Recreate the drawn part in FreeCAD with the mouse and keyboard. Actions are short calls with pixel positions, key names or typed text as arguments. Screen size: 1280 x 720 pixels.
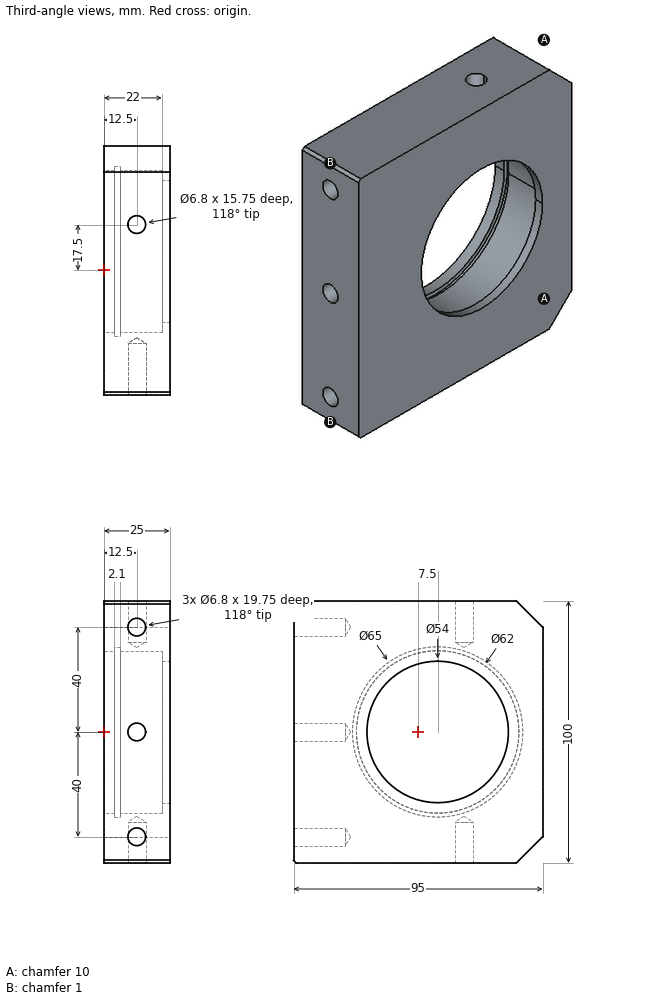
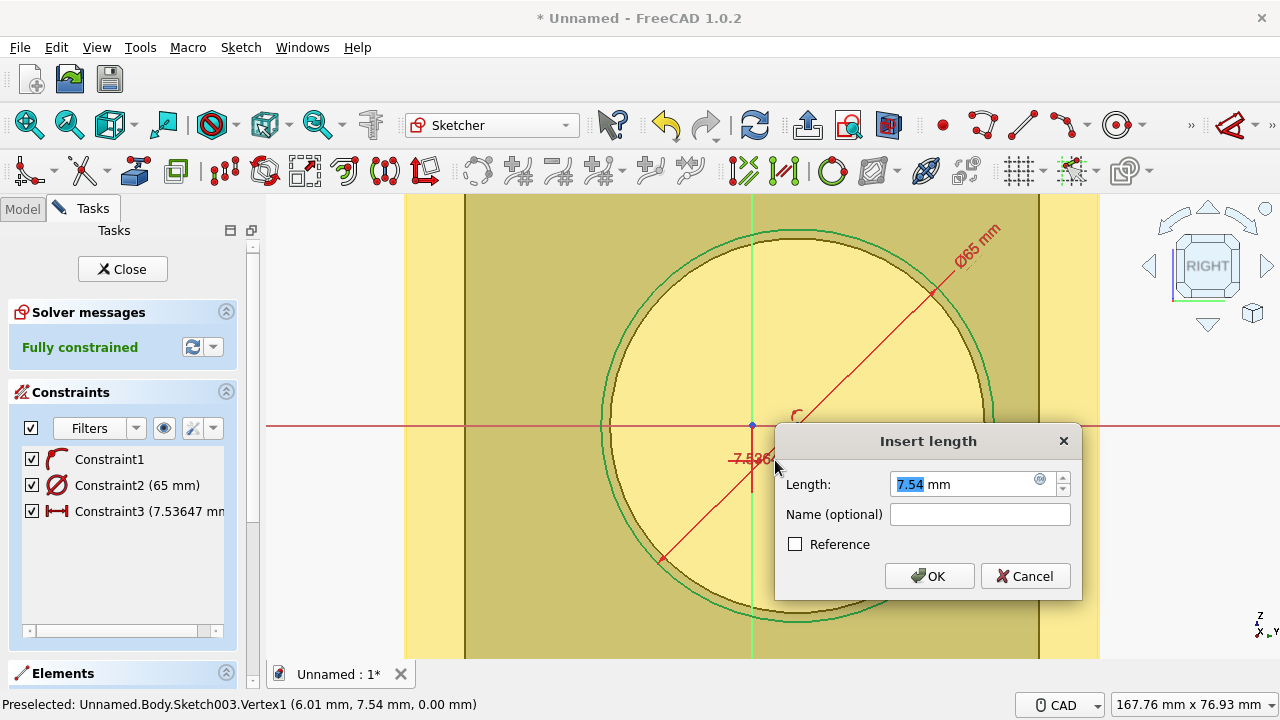
text(7.5)
key(Return)
key(Escape)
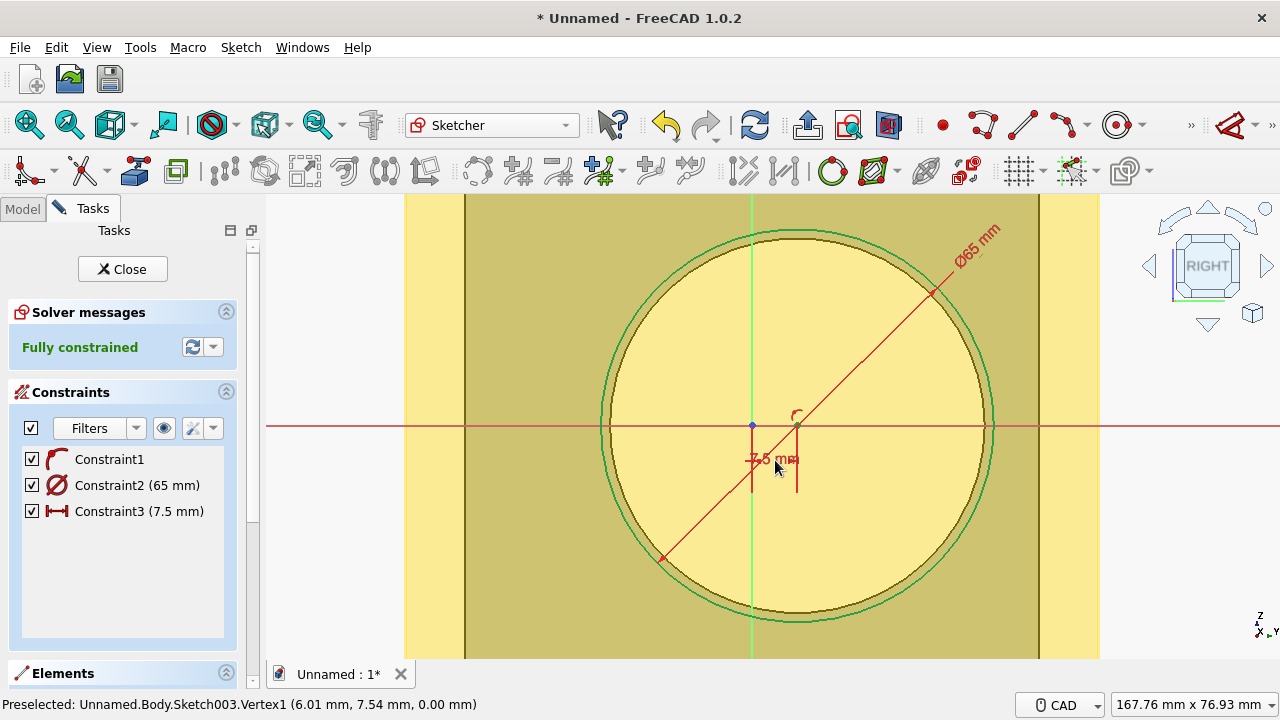
click(123, 269)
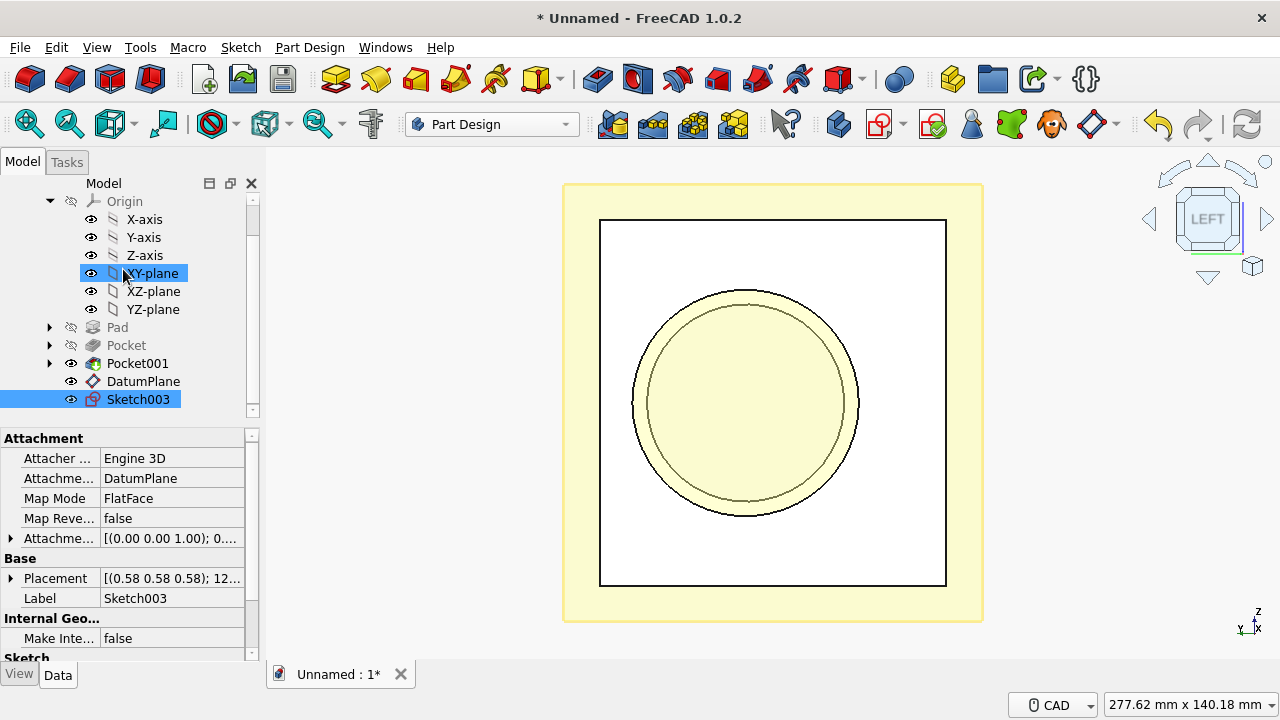
click(598, 80)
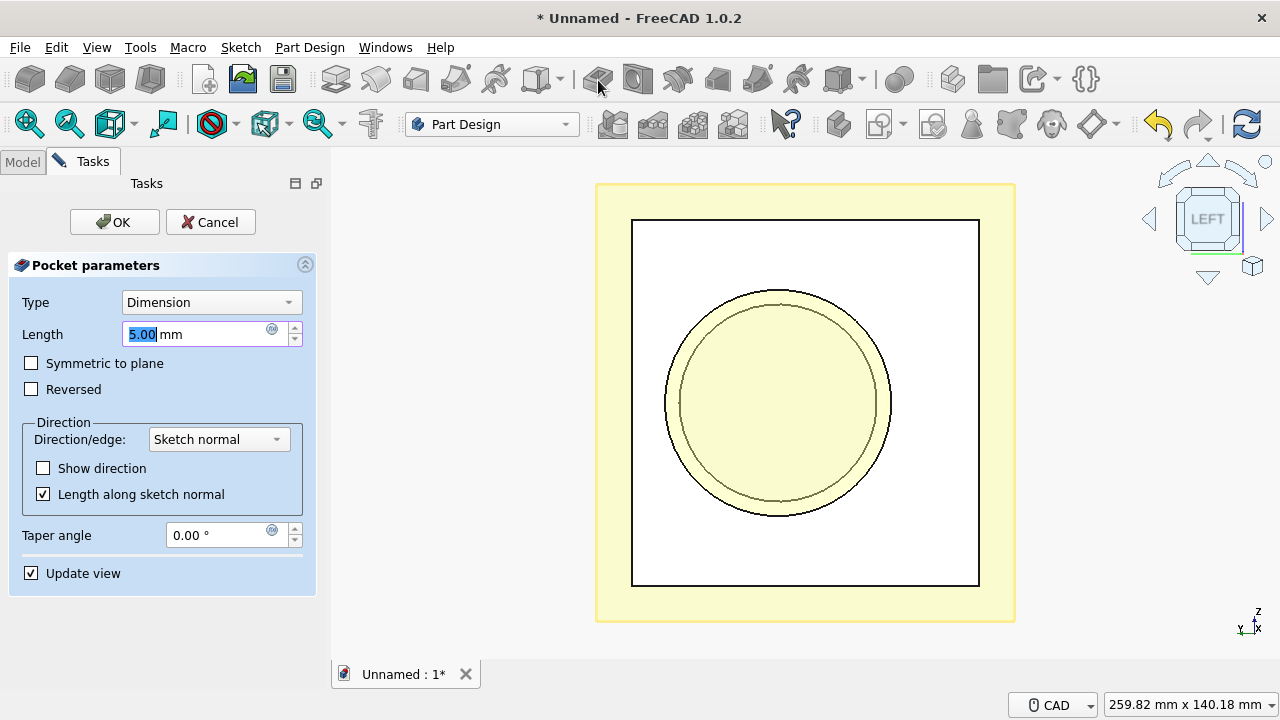
text(2.1)
key(Tab)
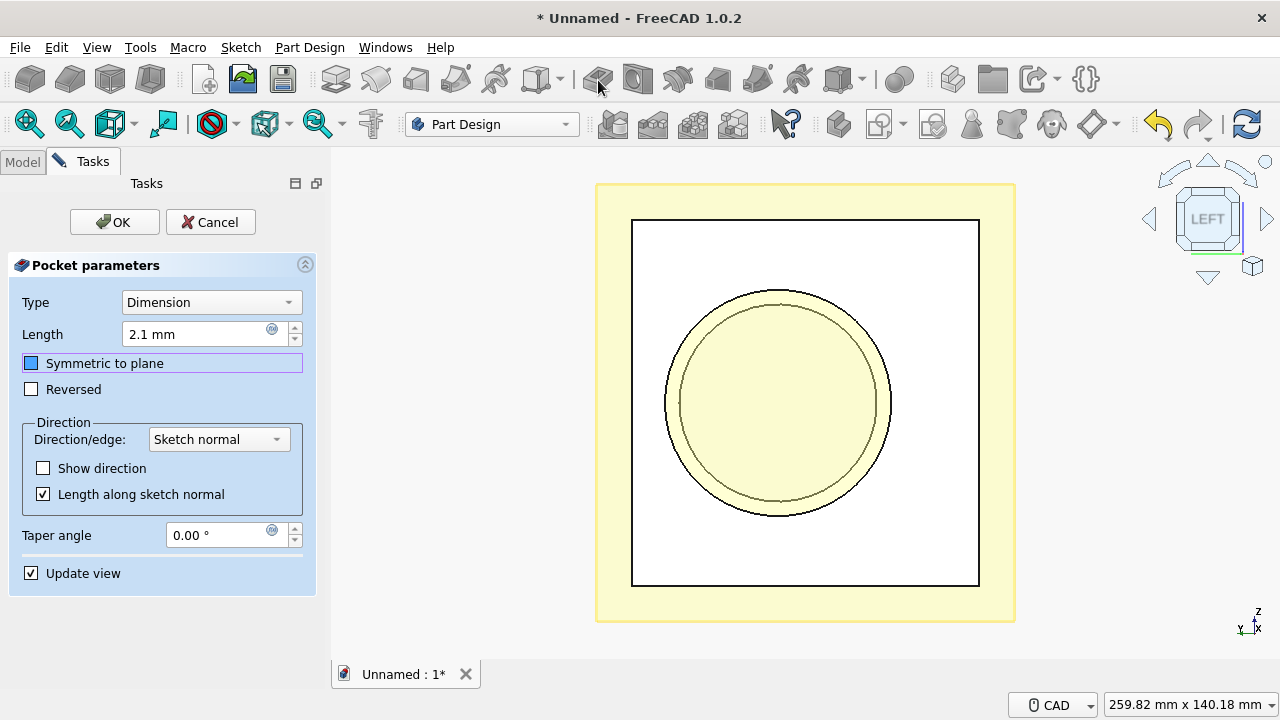
click(115, 222)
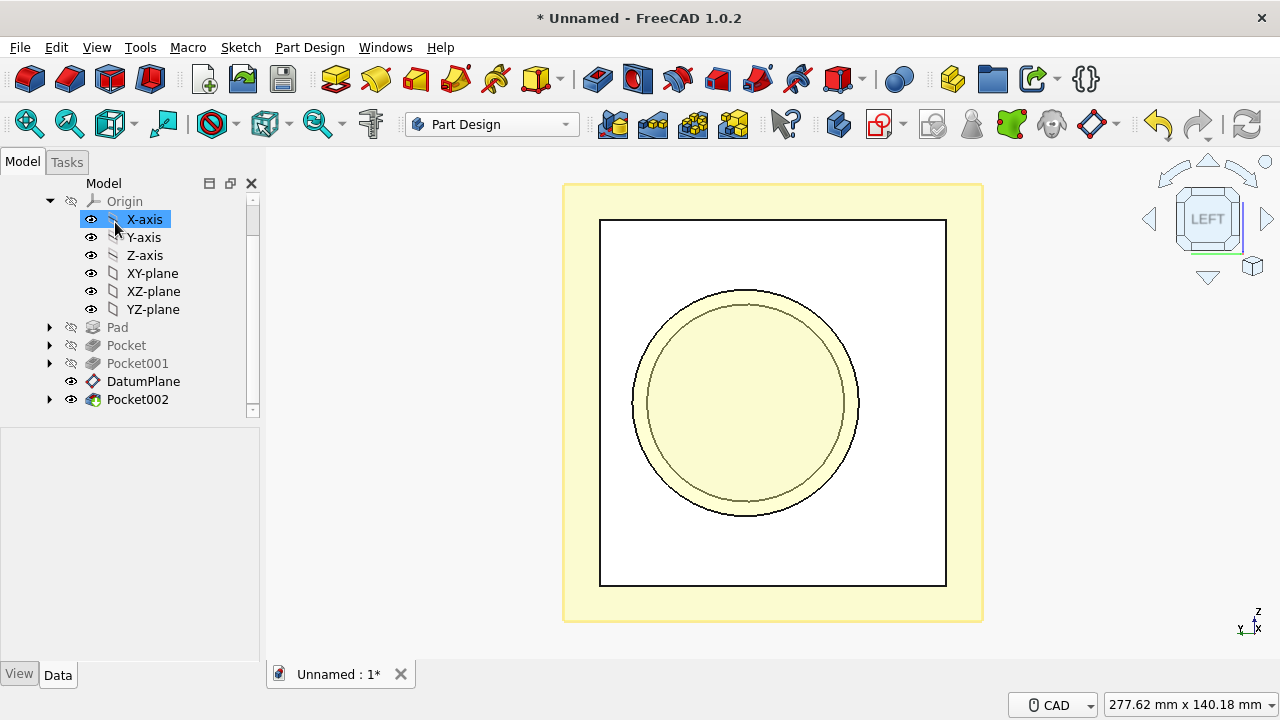
click(116, 381)
key(space)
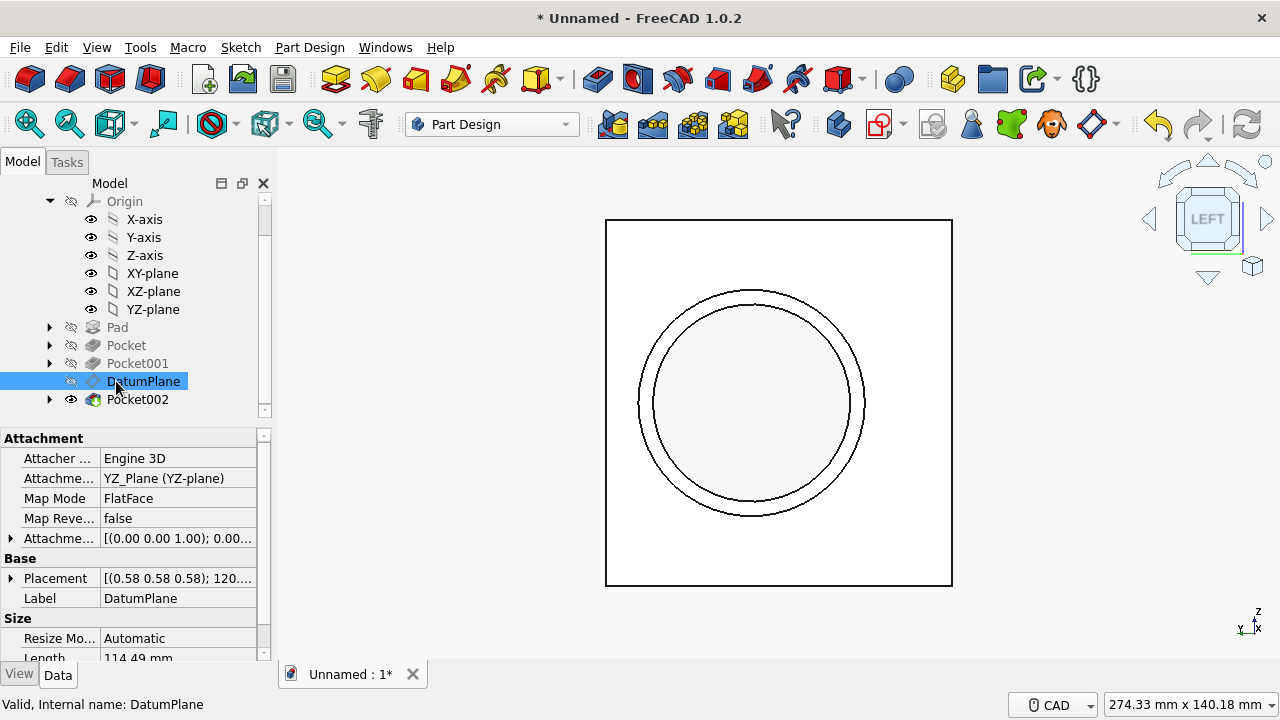
key(0)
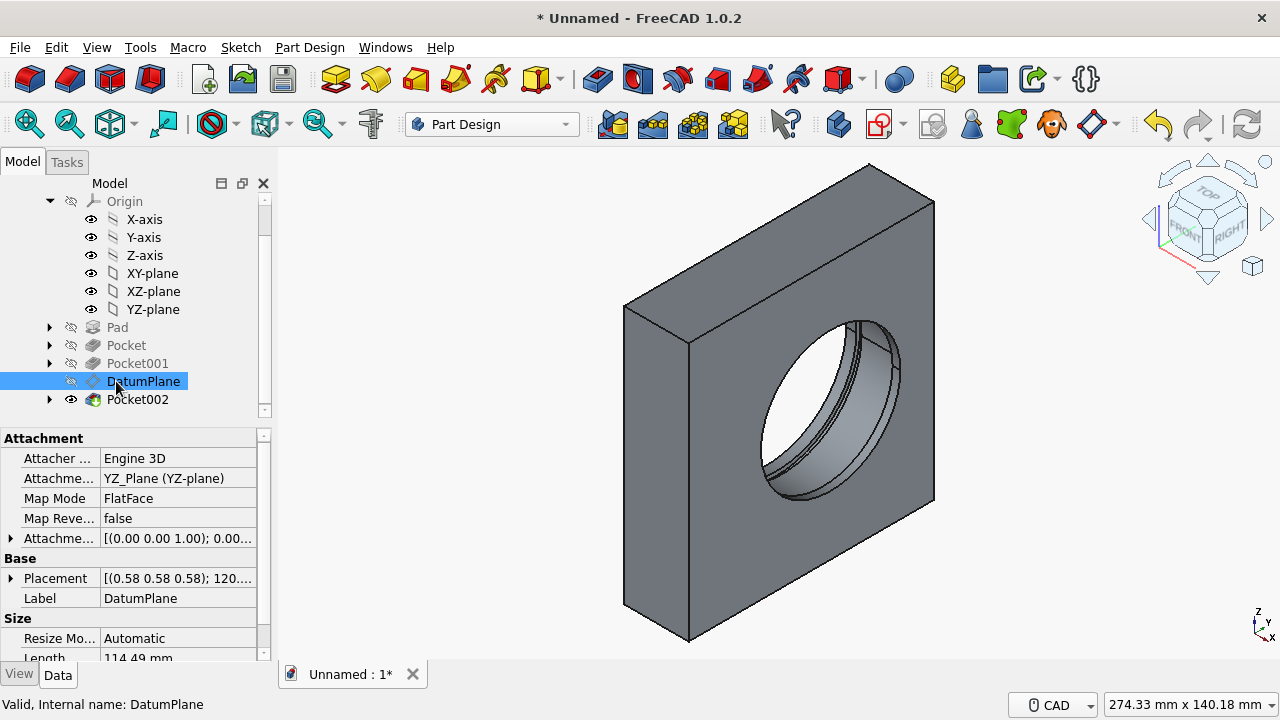
click(849, 212)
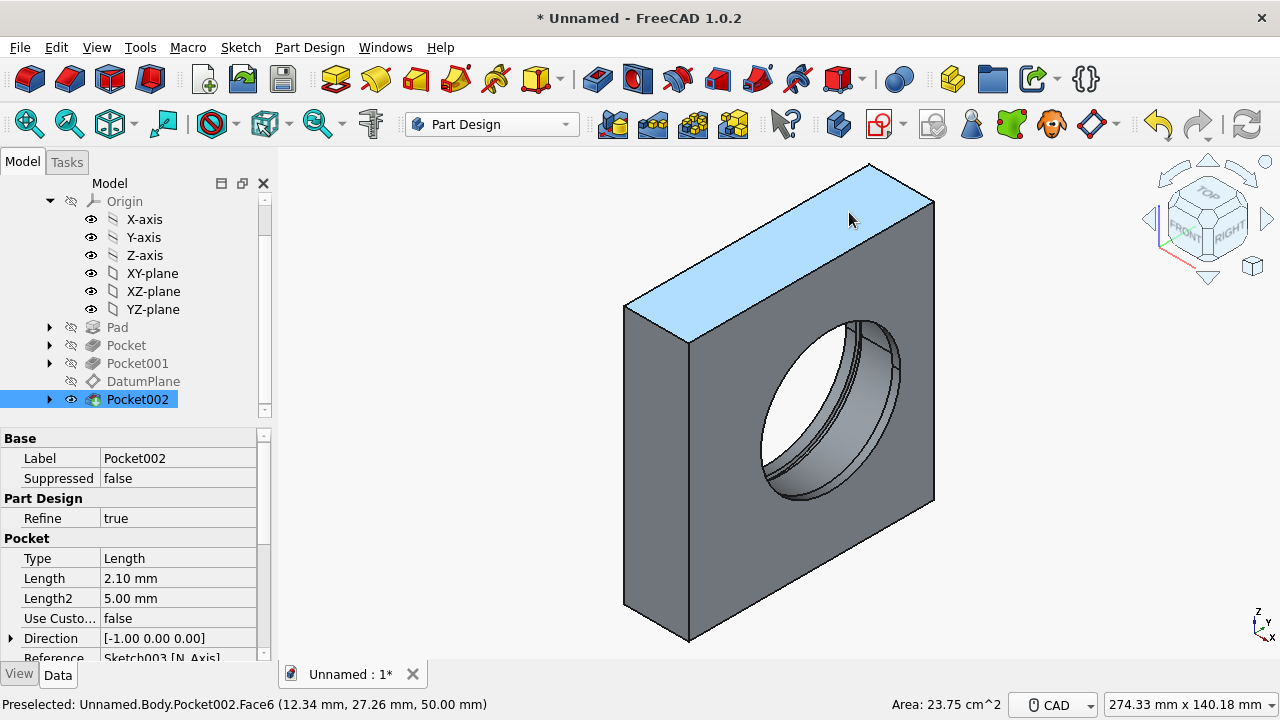
click(880, 124)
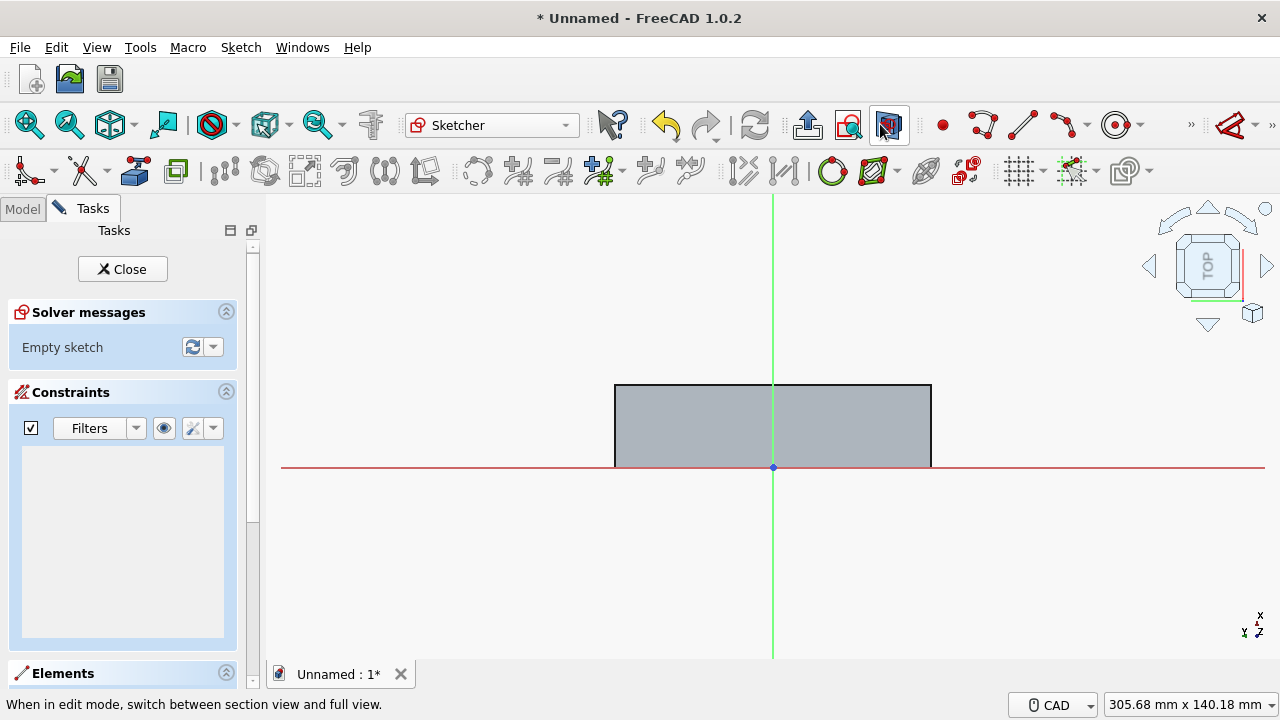
scroll(716, 427, up, 13)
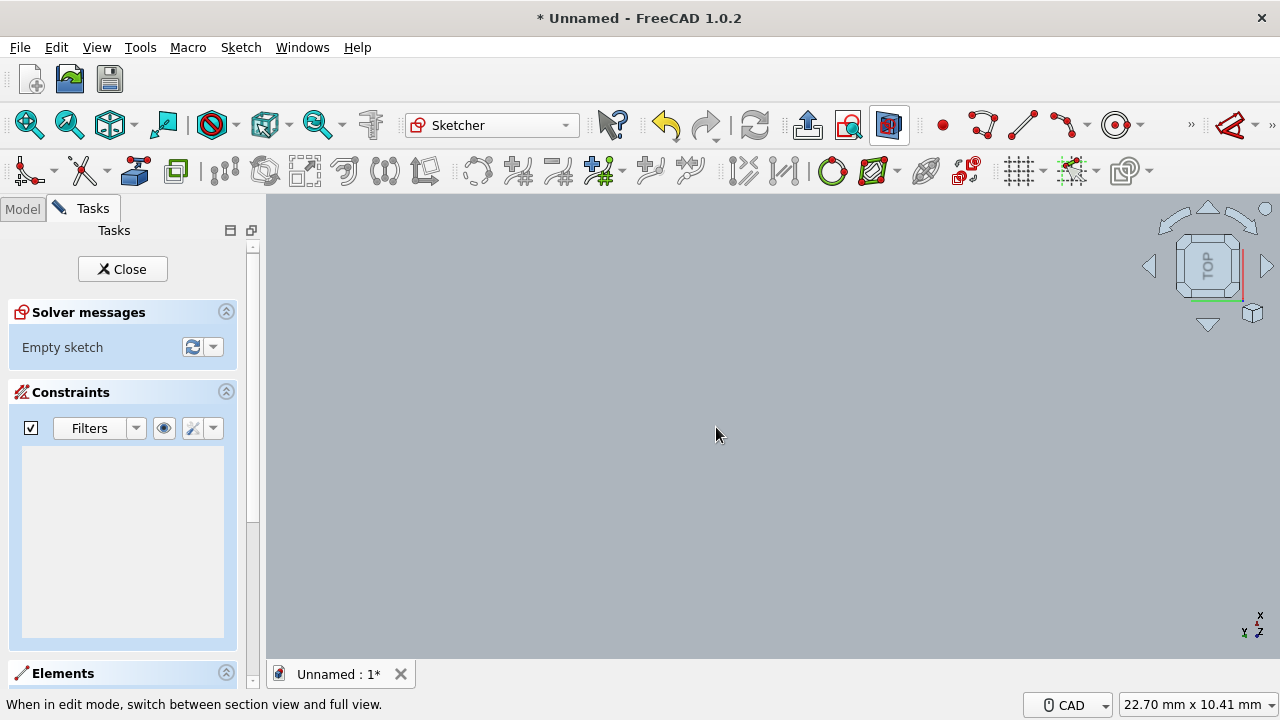
click(1116, 126)